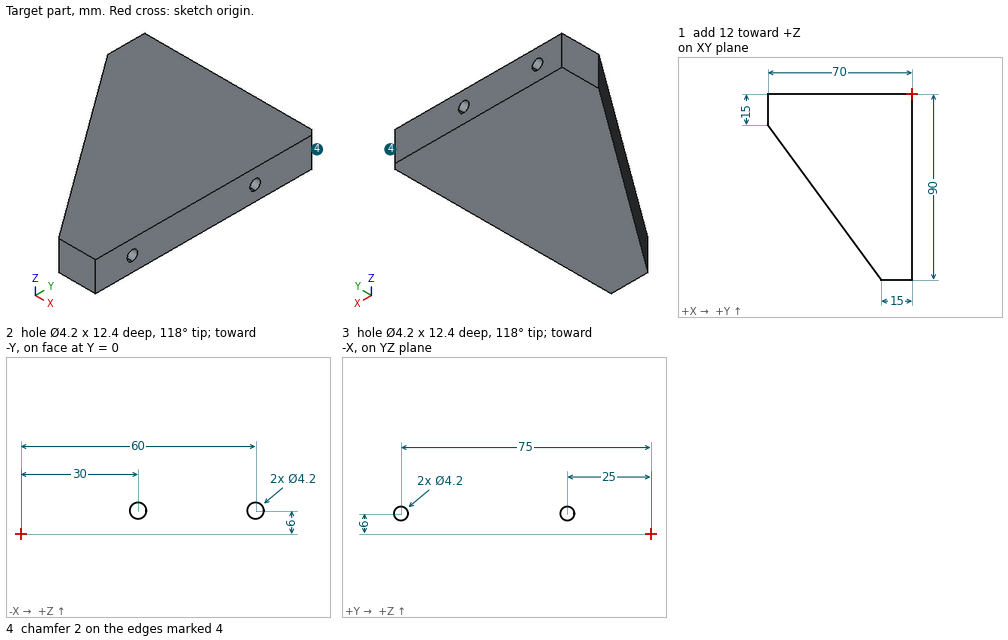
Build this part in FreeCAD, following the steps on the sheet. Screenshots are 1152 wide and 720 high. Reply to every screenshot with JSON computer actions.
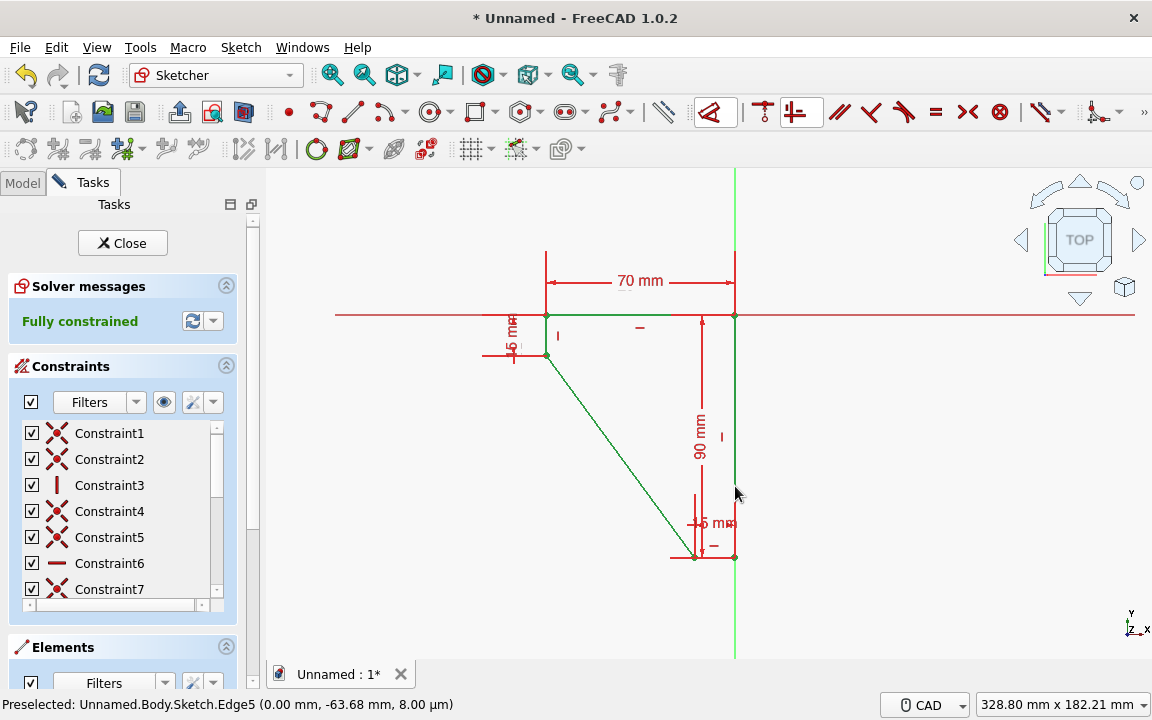
{"action": "left_click", "coordinate": [123, 243]}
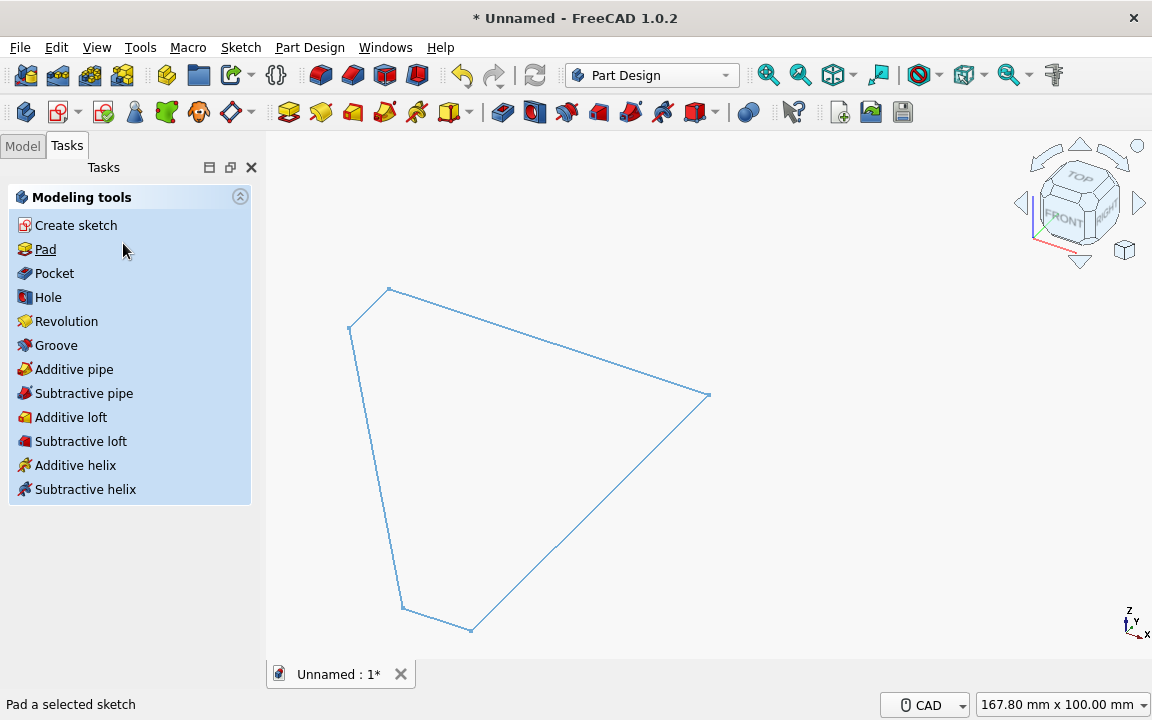
{"action": "left_click", "coordinate": [290, 112]}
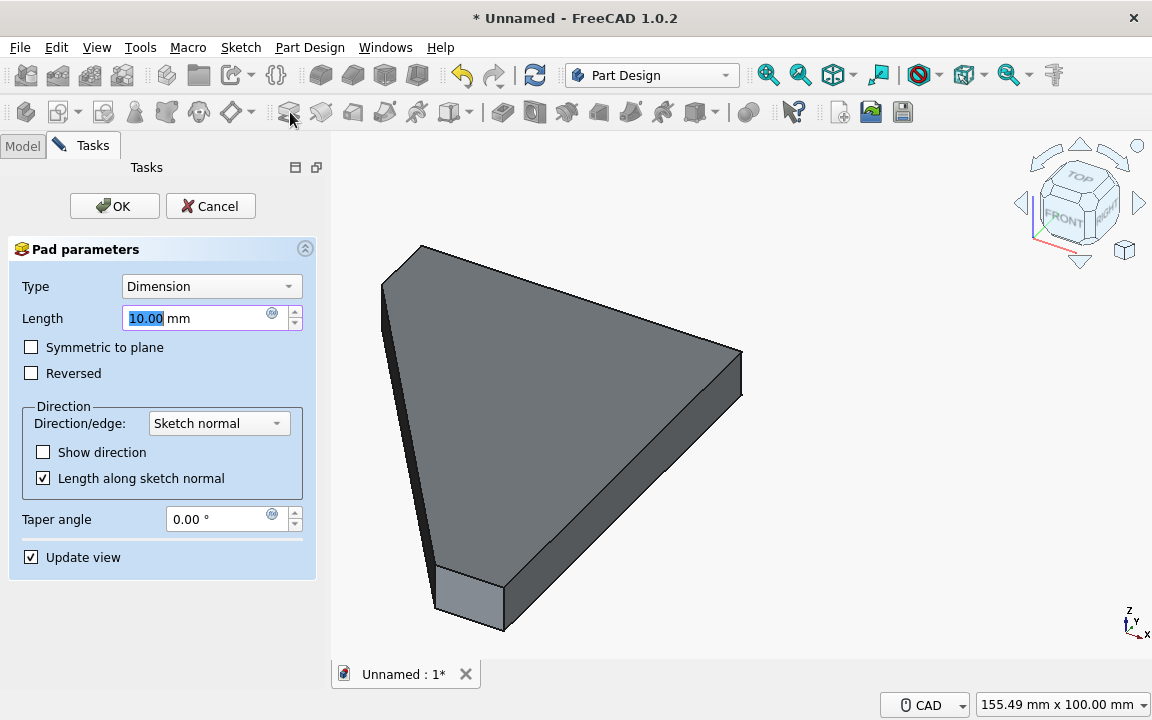
{"action": "type", "text": "12"}
{"action": "key", "text": "Tab"}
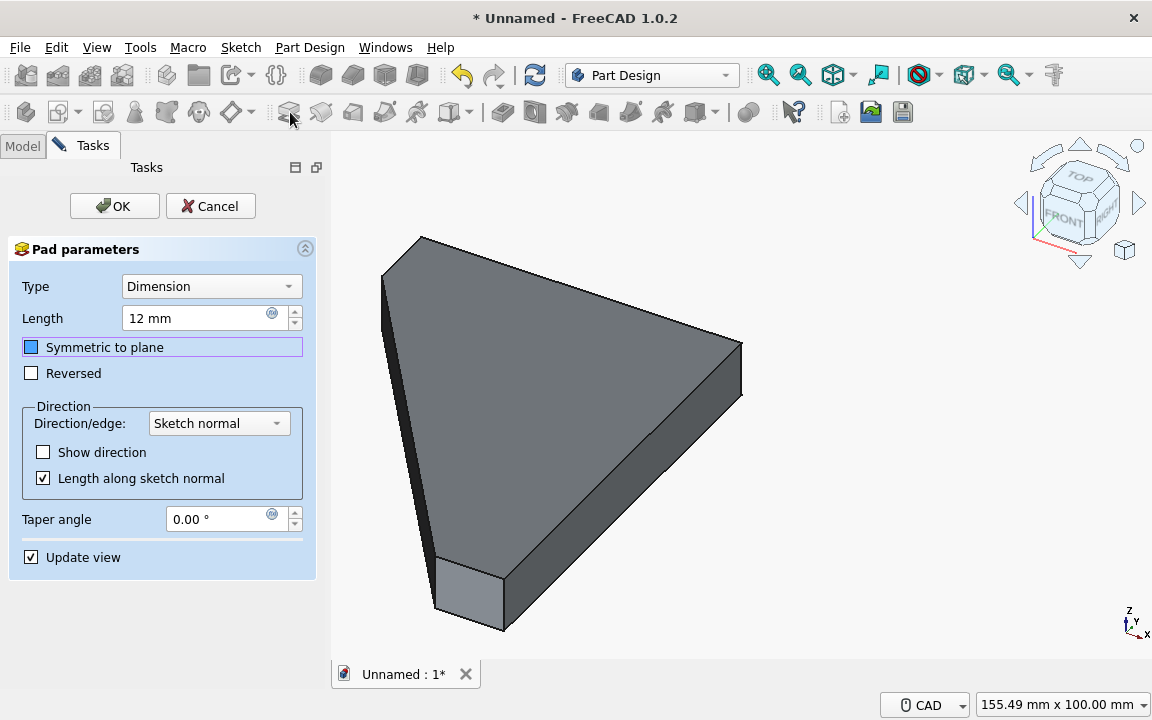
{"action": "left_click", "coordinate": [115, 206]}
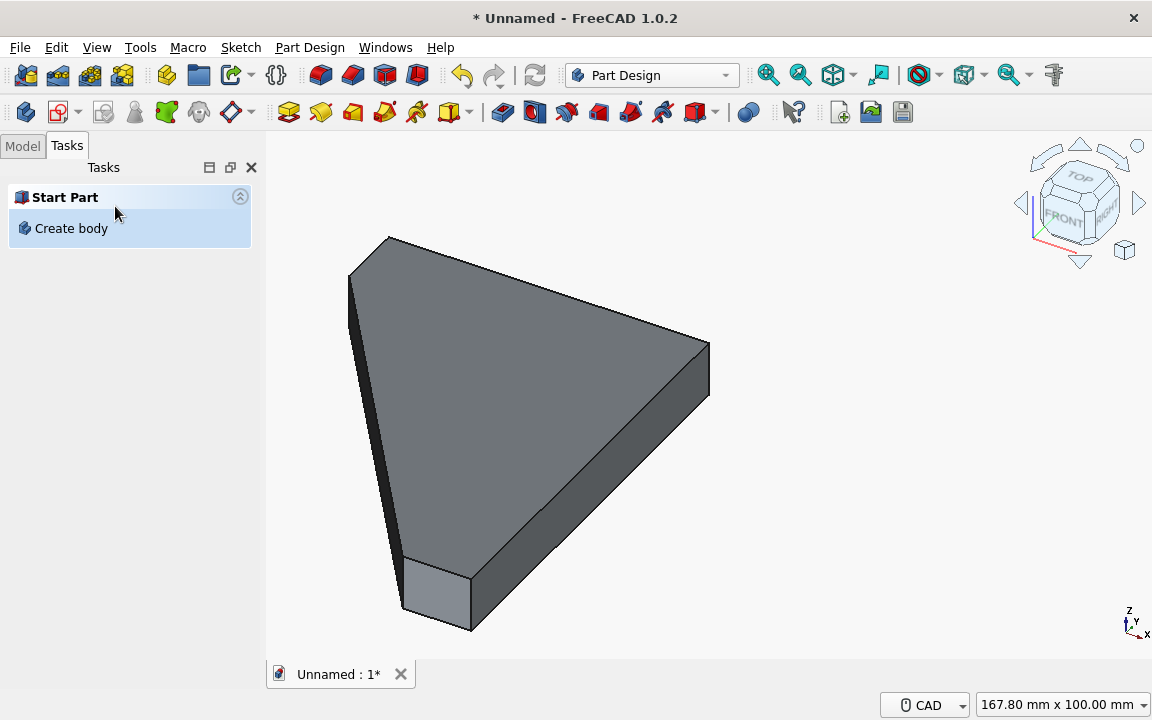
{"action": "key", "text": "v f"}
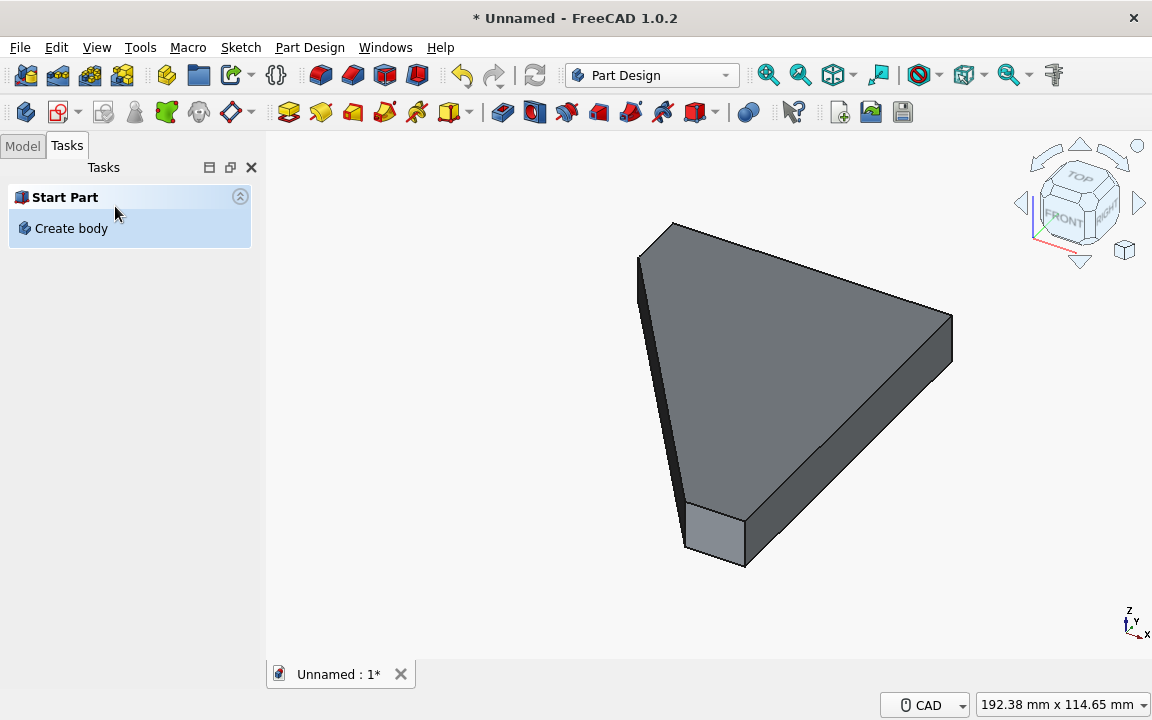
{"action": "key", "text": "4"}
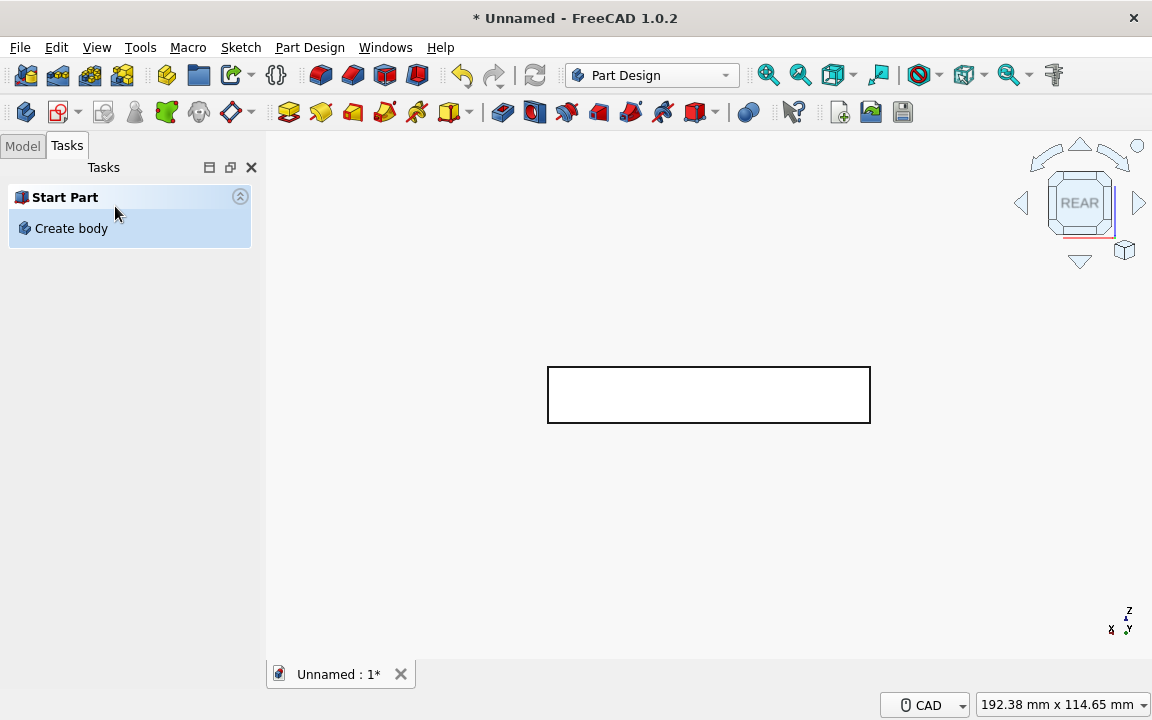
{"action": "left_click", "coordinate": [770, 76]}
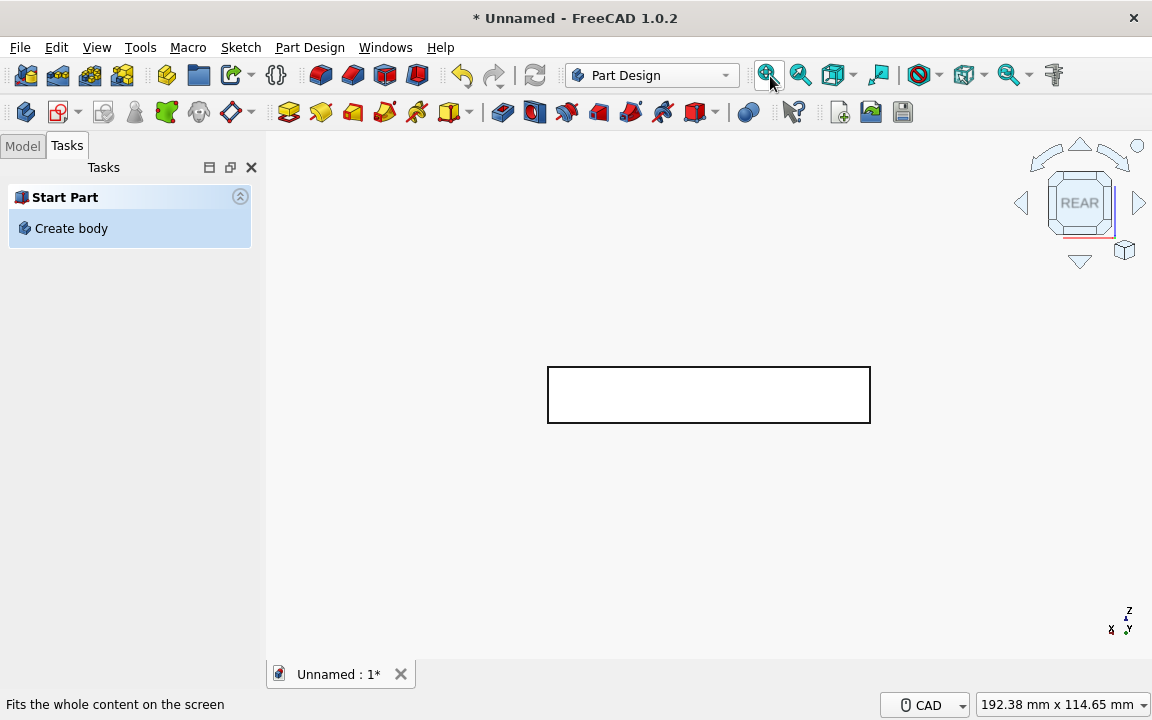
{"action": "left_click", "coordinate": [617, 394]}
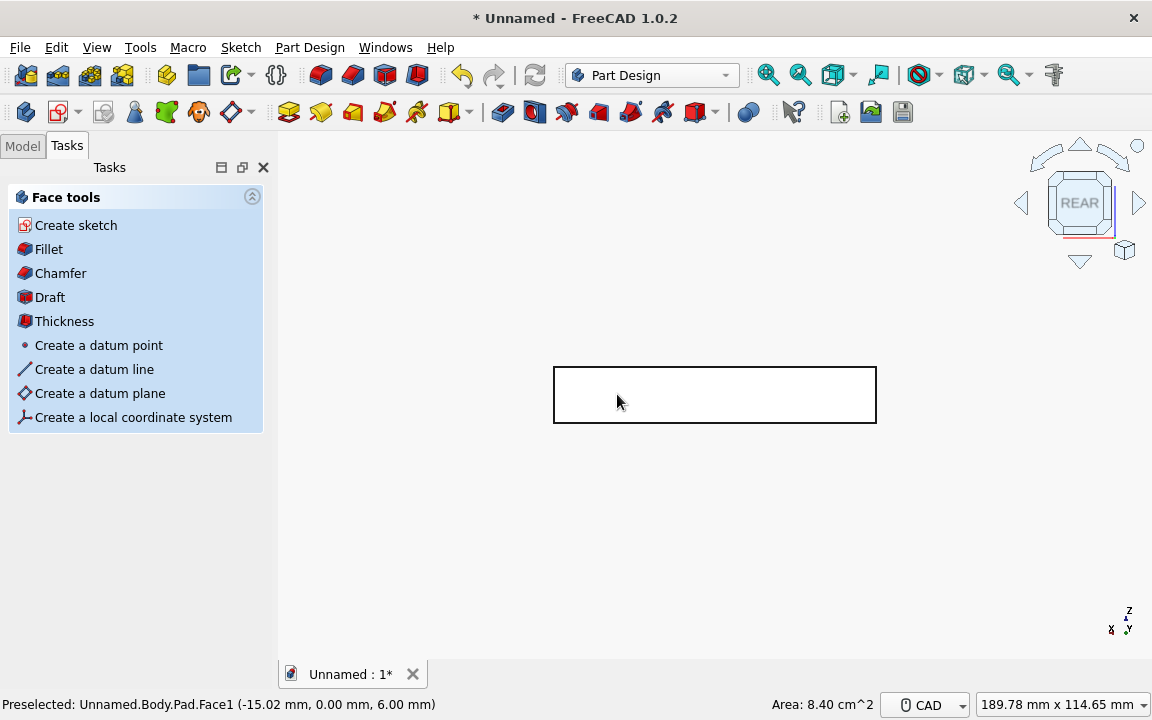
{"action": "left_click", "coordinate": [58, 112]}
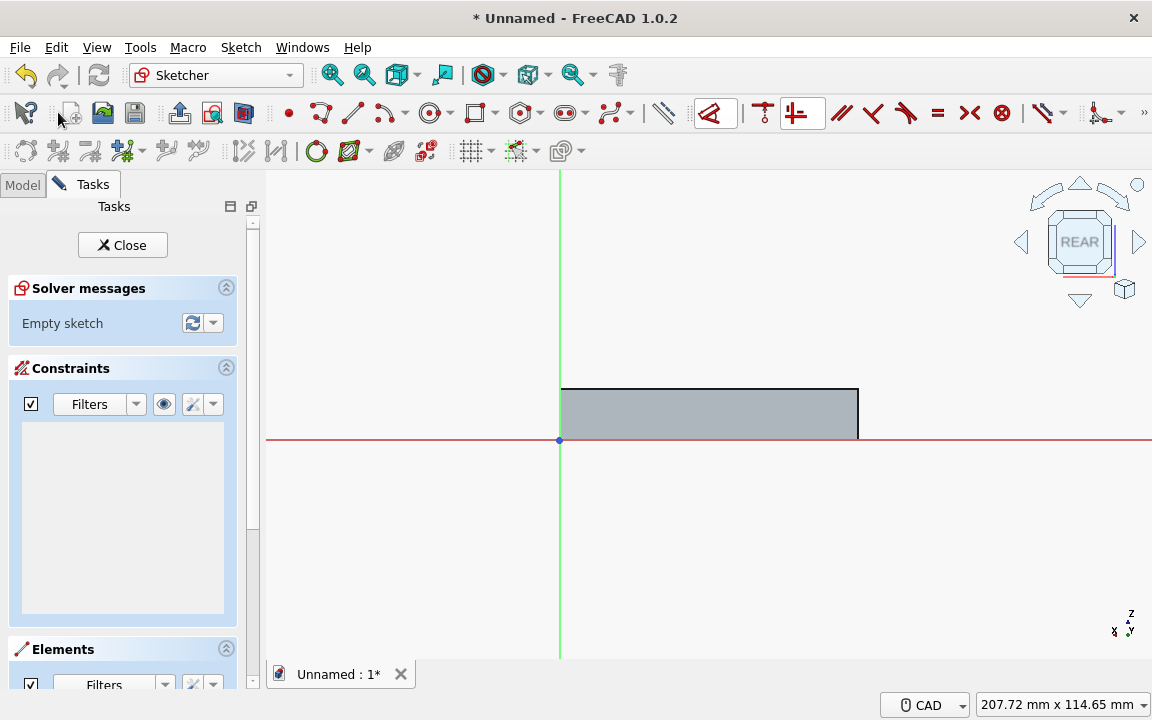
{"action": "scroll", "coordinate": [755, 433], "scroll_direction": "up", "scroll_amount": 3}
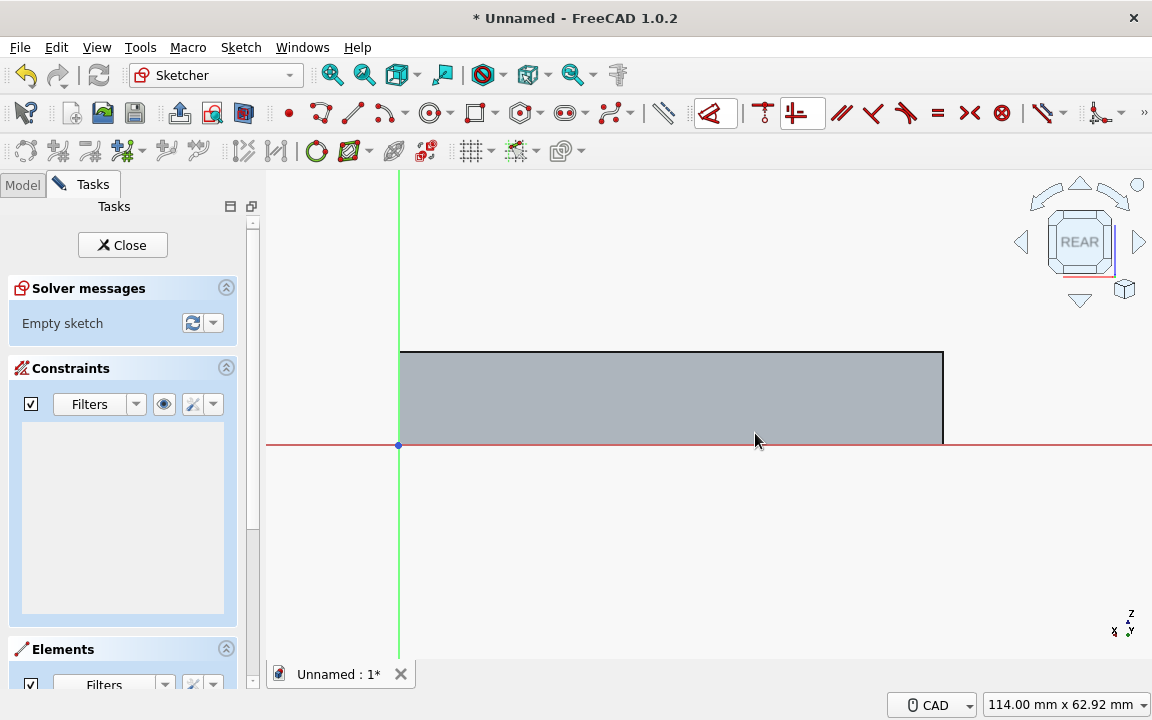
{"action": "key", "text": "g c"}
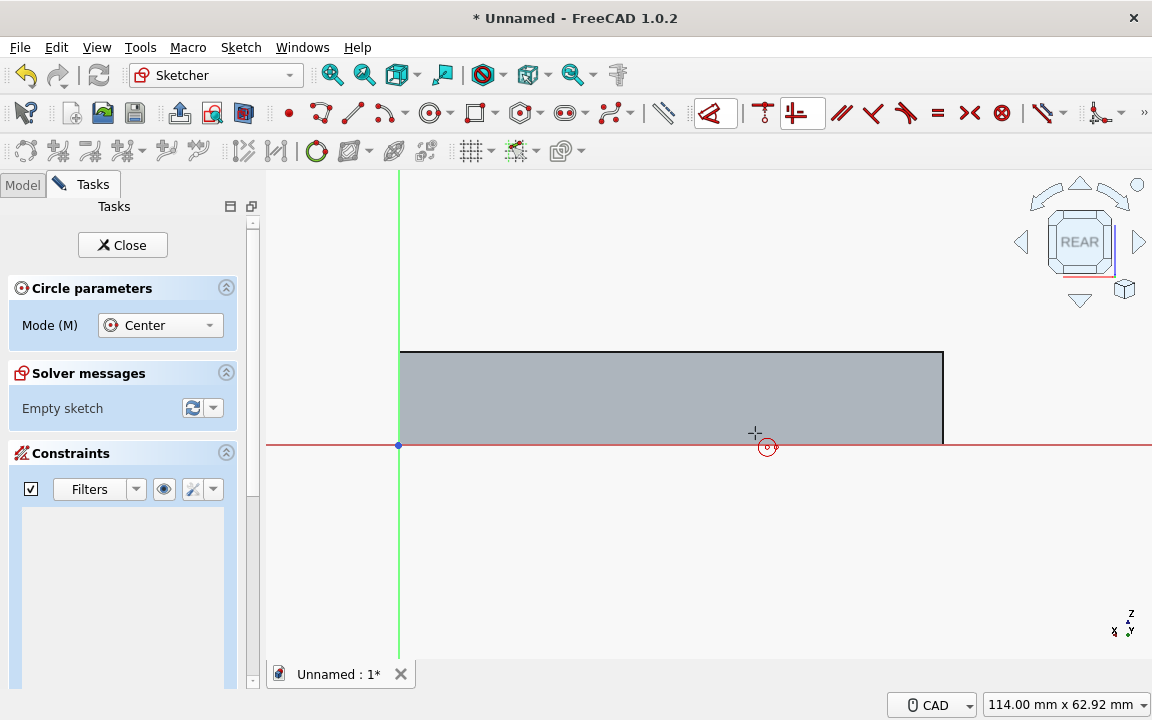
{"action": "scroll", "coordinate": [865, 399], "scroll_direction": "up", "scroll_amount": 2}